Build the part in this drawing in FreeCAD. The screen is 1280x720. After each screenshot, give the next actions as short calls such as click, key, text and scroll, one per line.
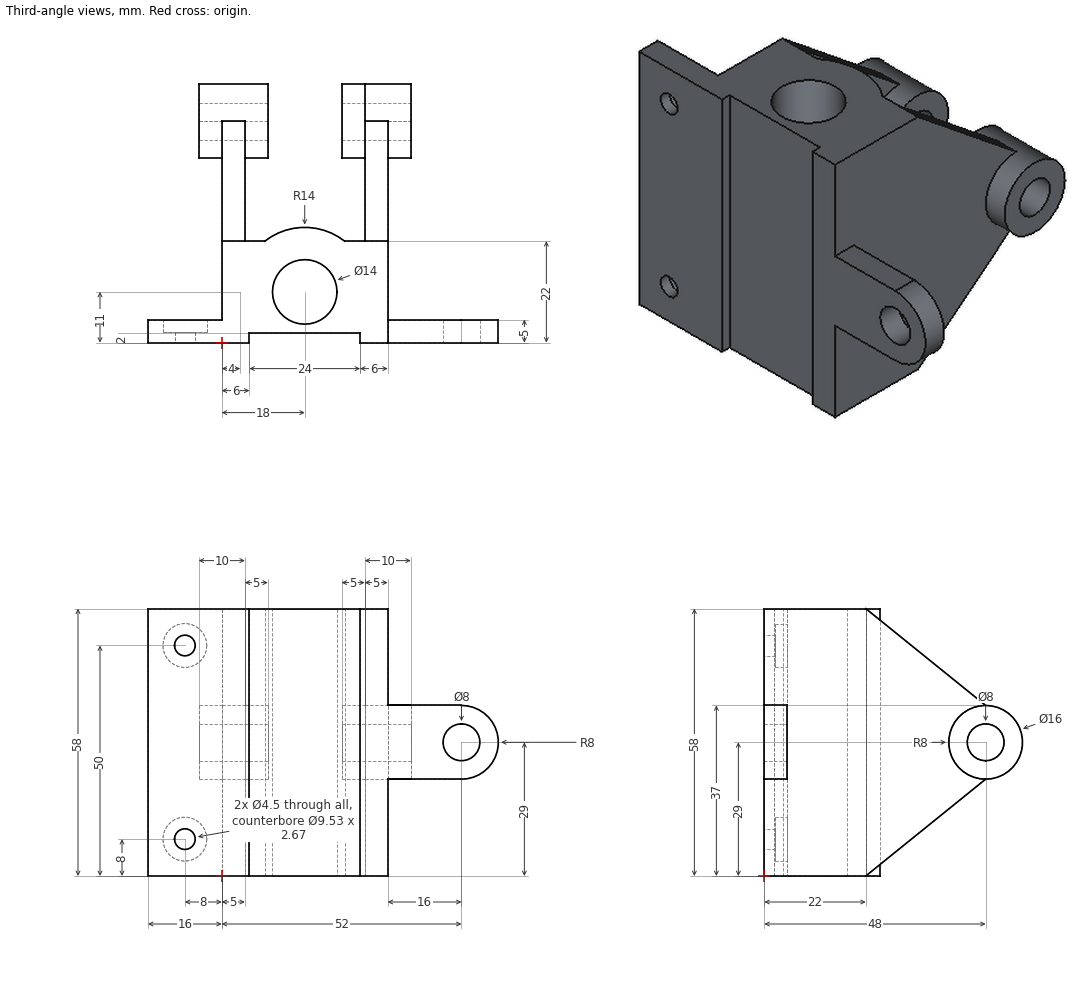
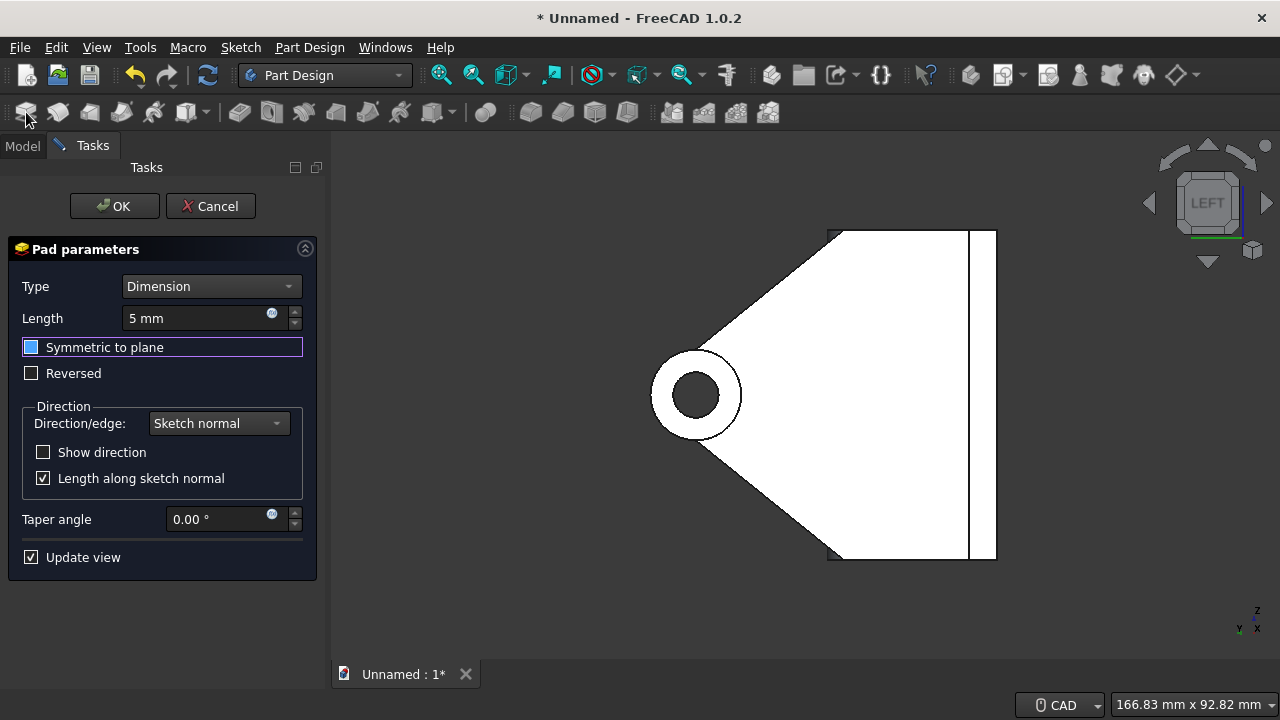
click(30, 373)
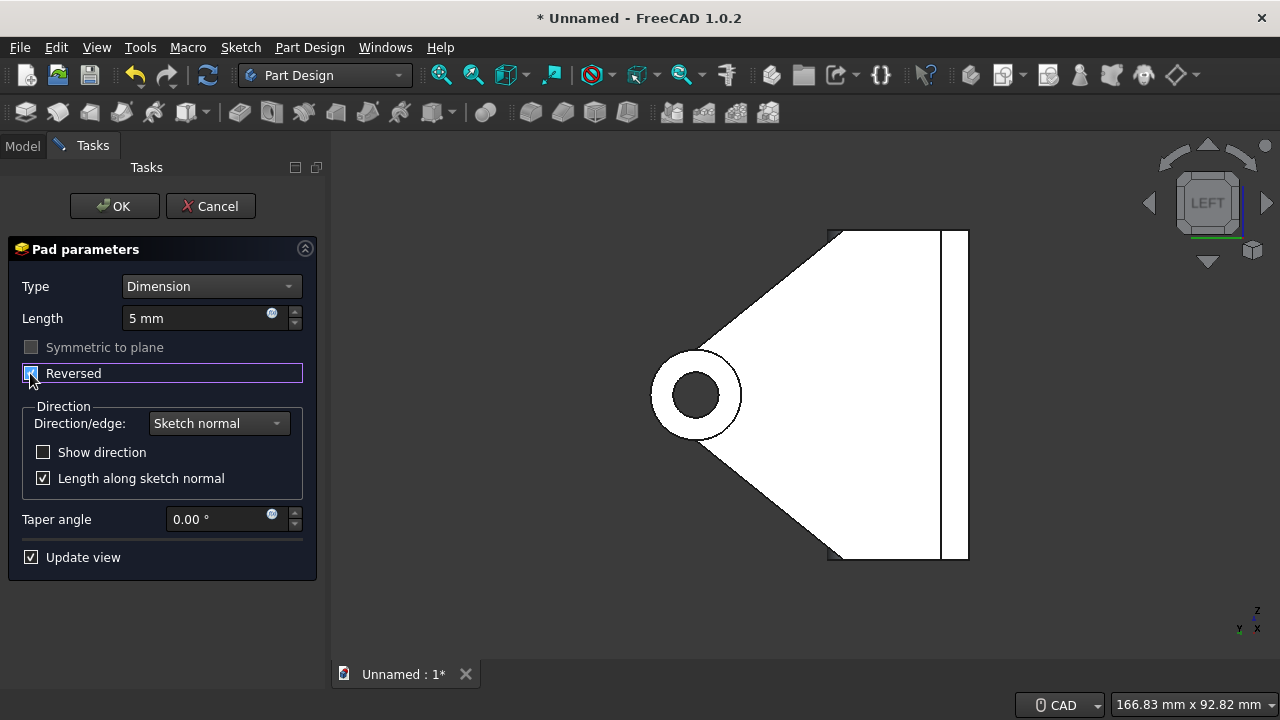
click(115, 206)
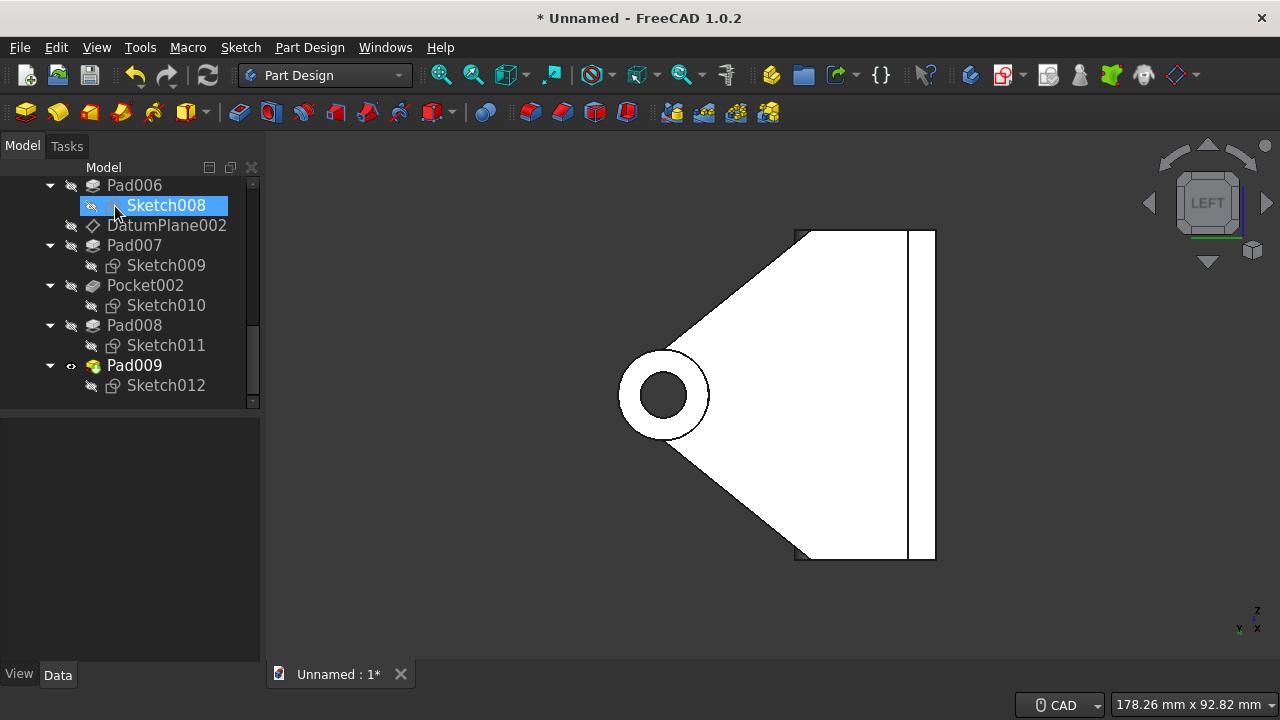
key(4)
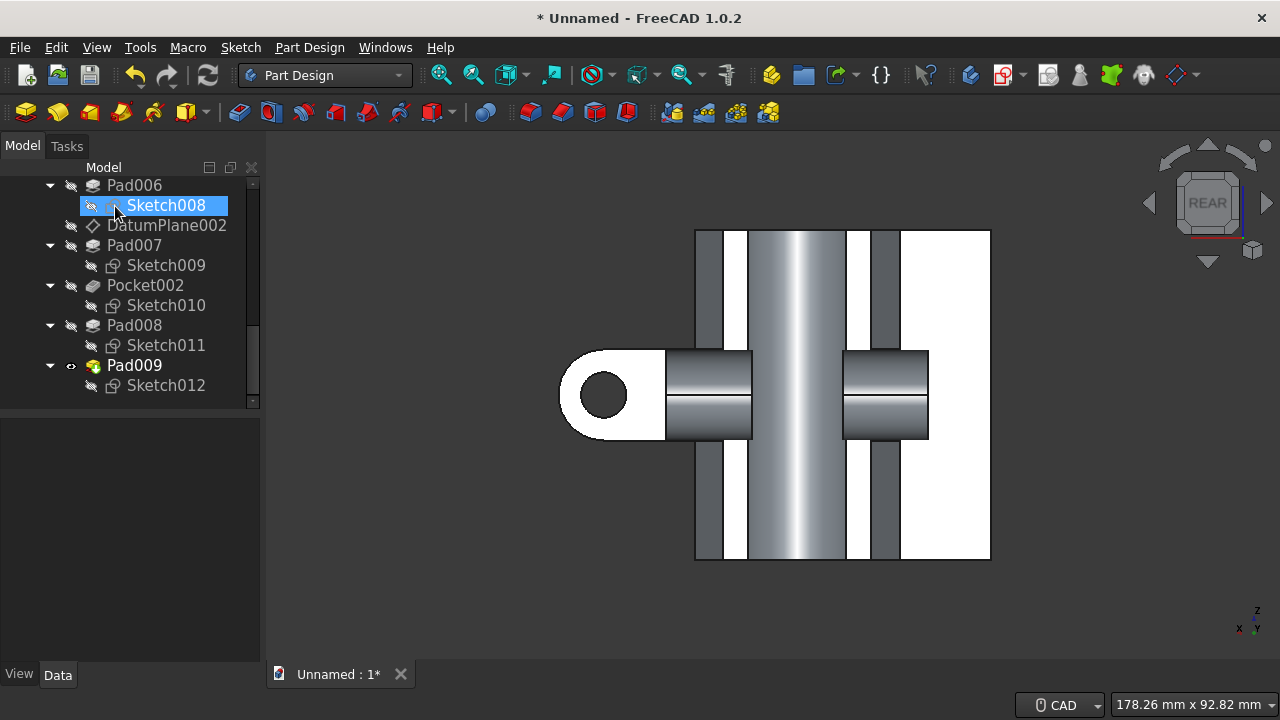
click(945, 300)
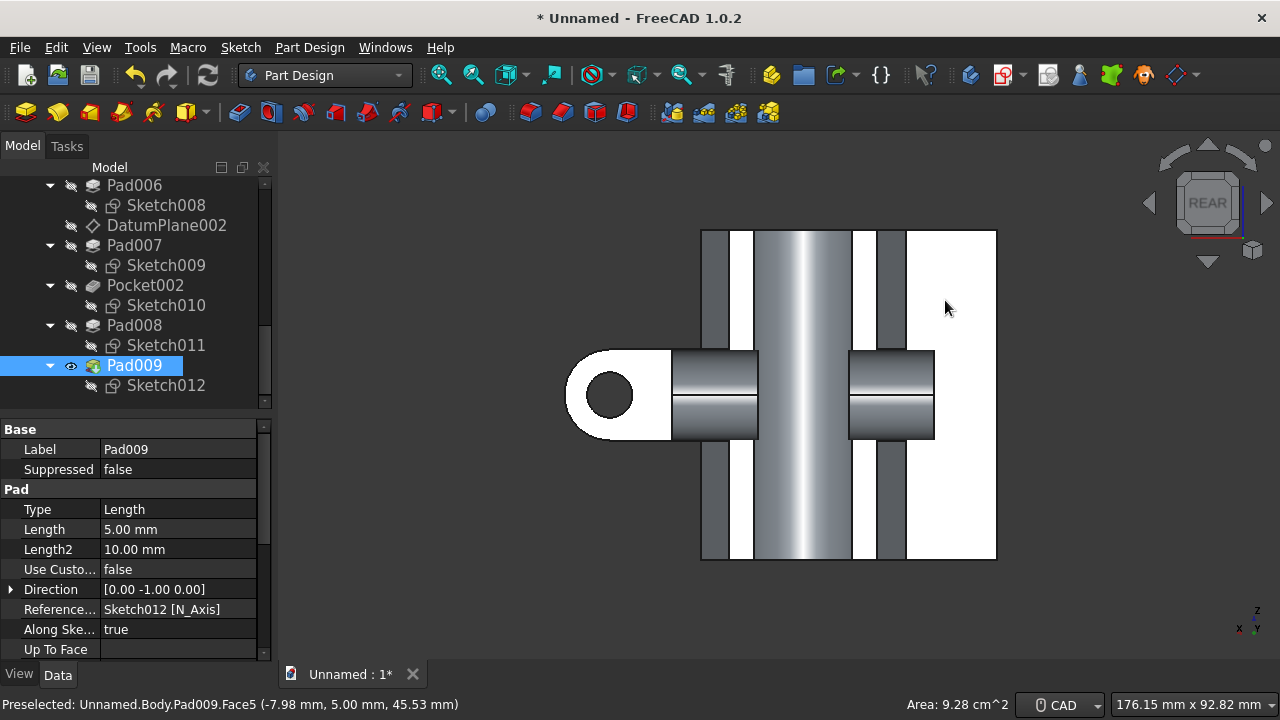
click(1004, 76)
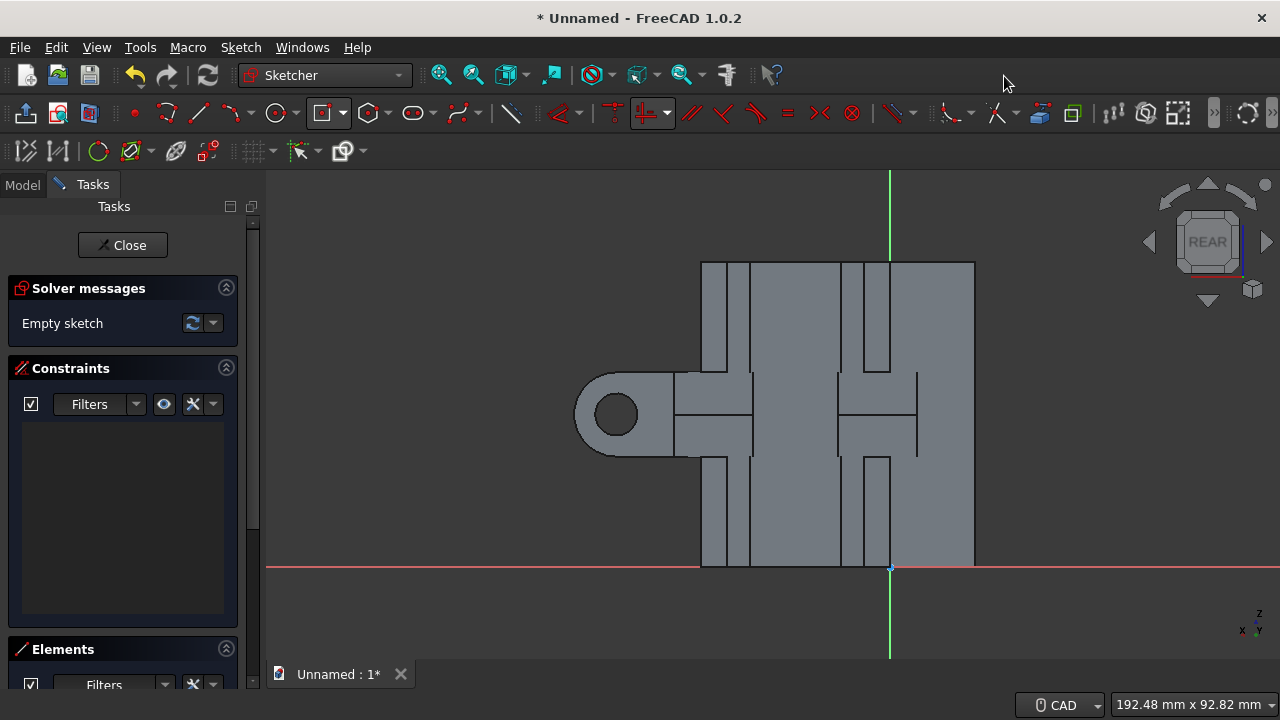
click(90, 114)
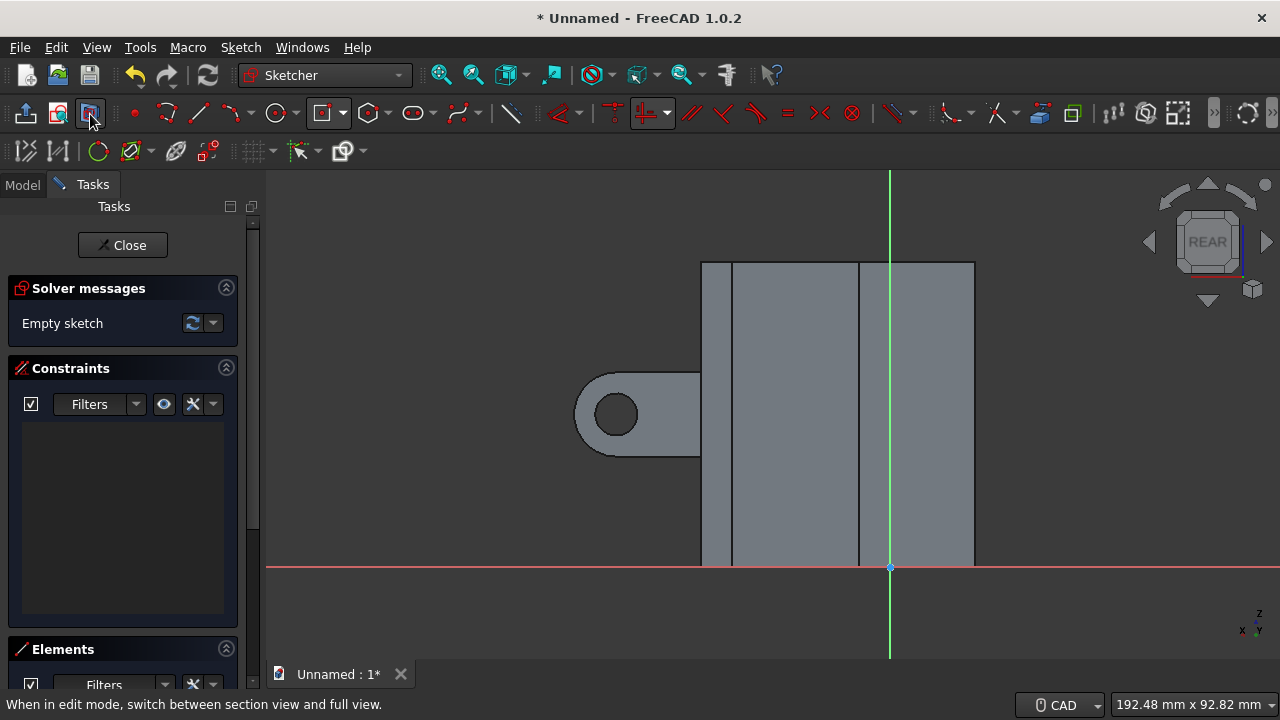
key(g)
key(c)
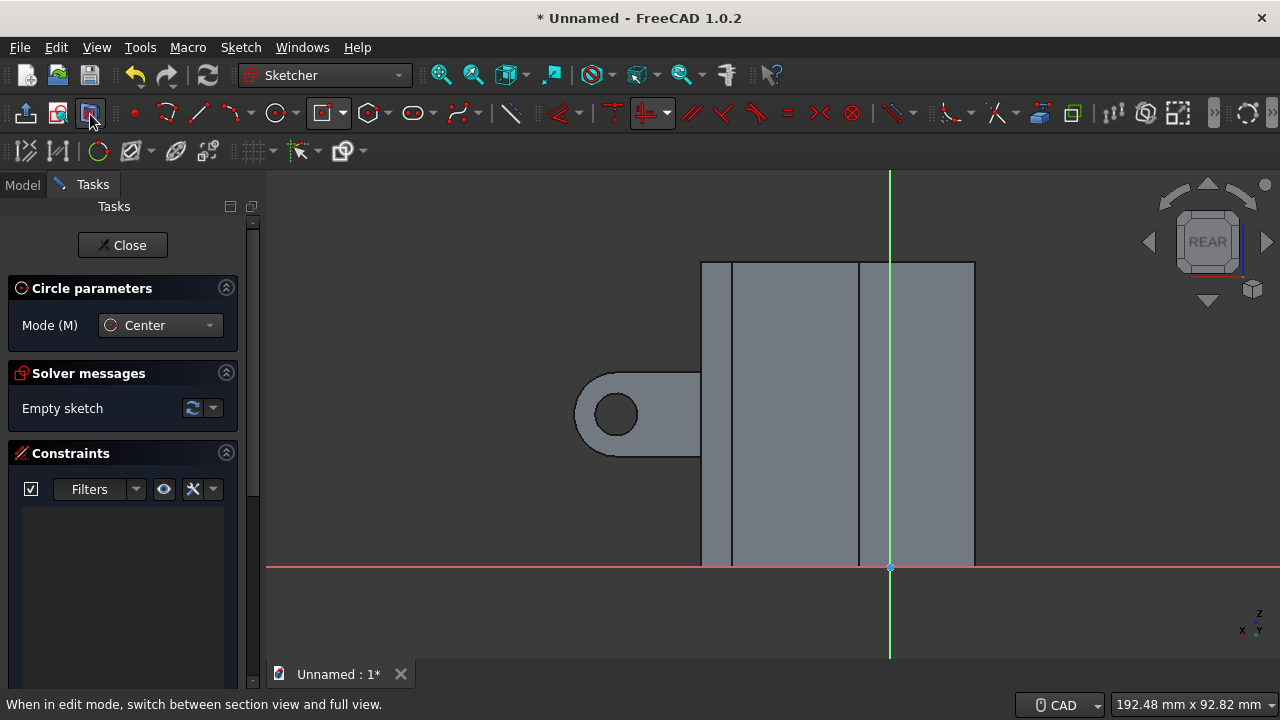
scroll(932, 525, up, 4)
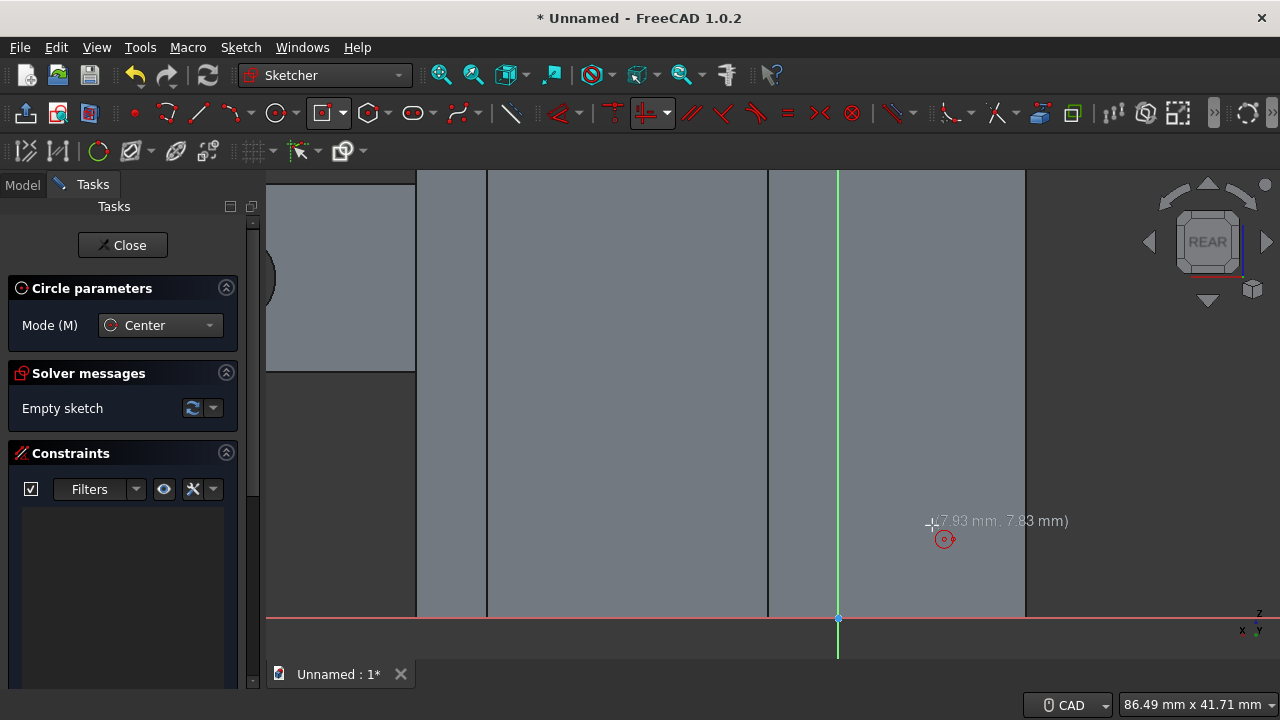
click(932, 524)
move(951, 506)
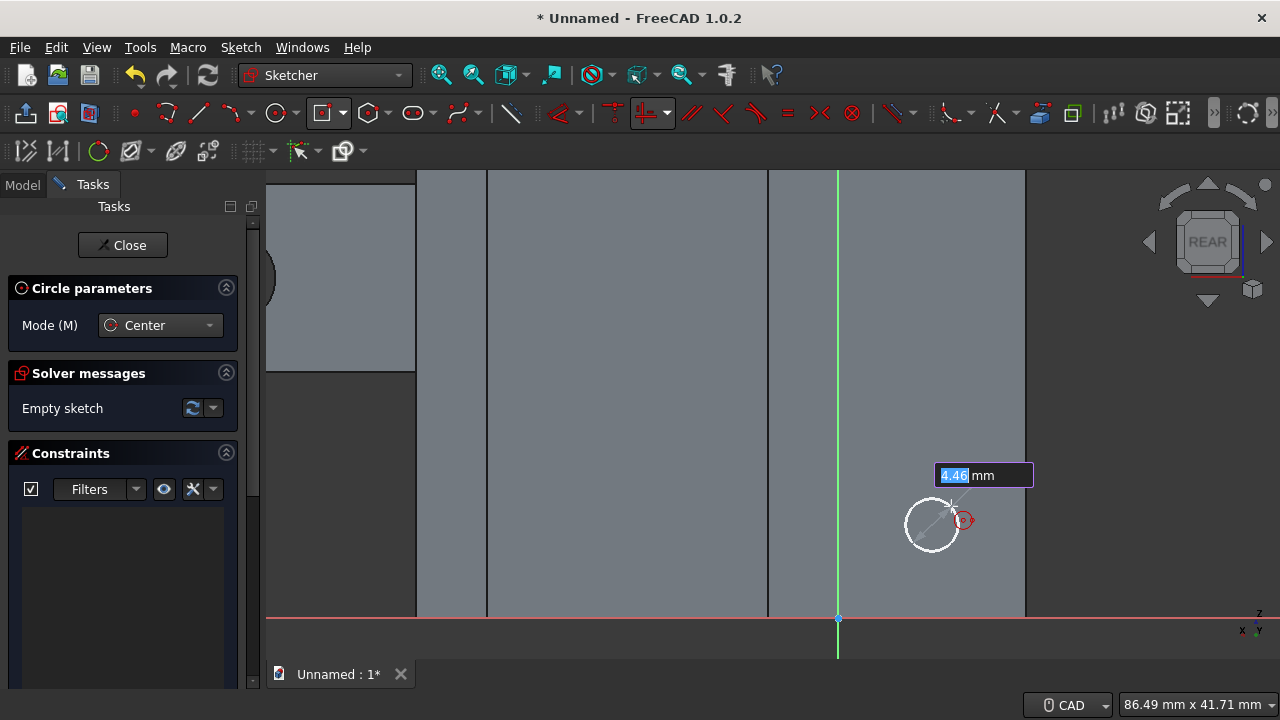
text(4.5)
key(Return)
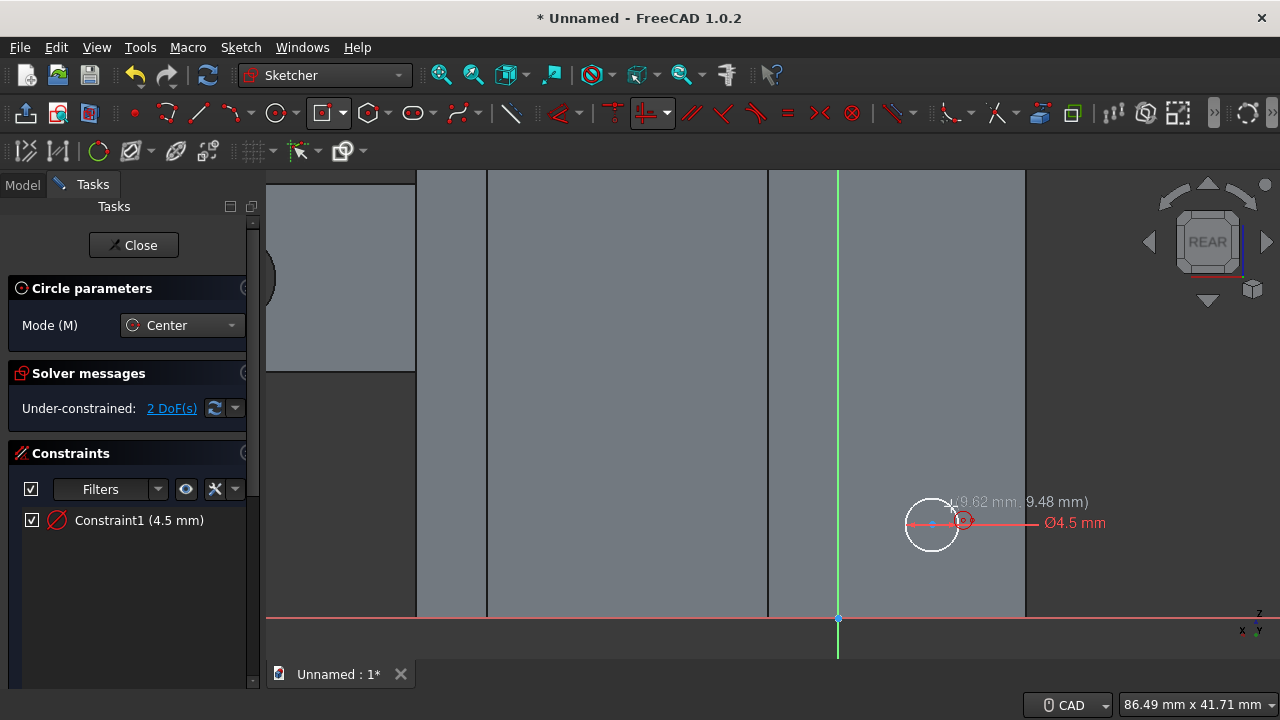
scroll(469, 539, down, 3)